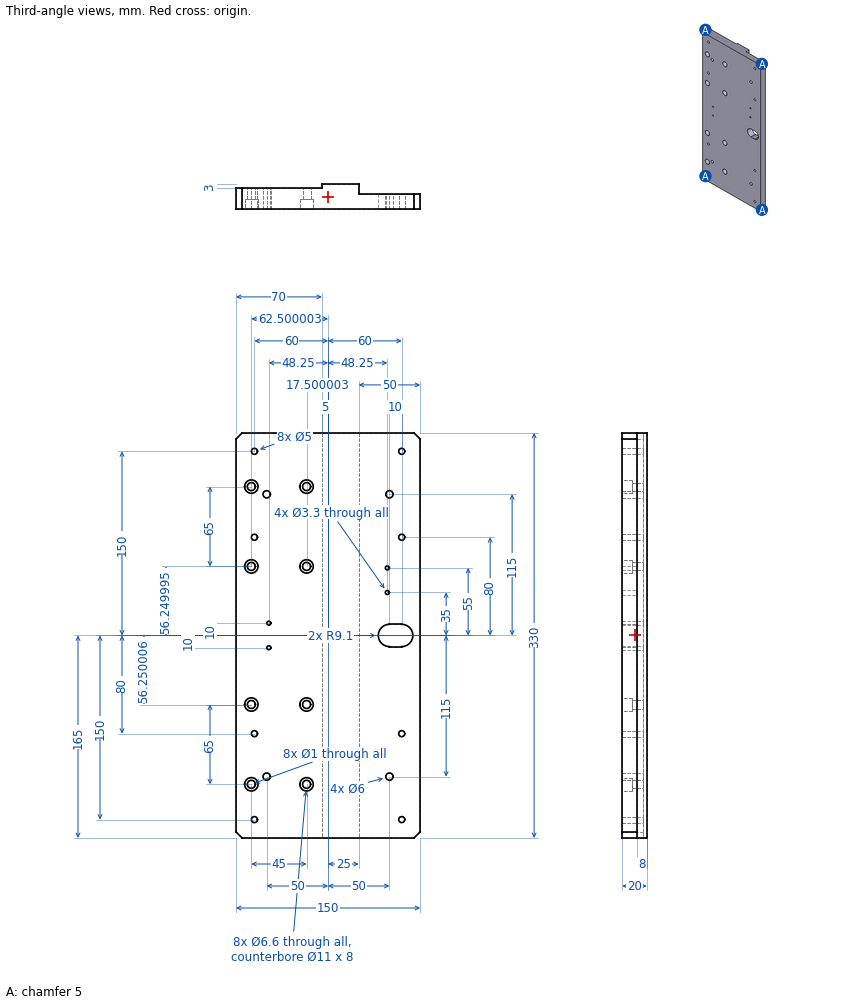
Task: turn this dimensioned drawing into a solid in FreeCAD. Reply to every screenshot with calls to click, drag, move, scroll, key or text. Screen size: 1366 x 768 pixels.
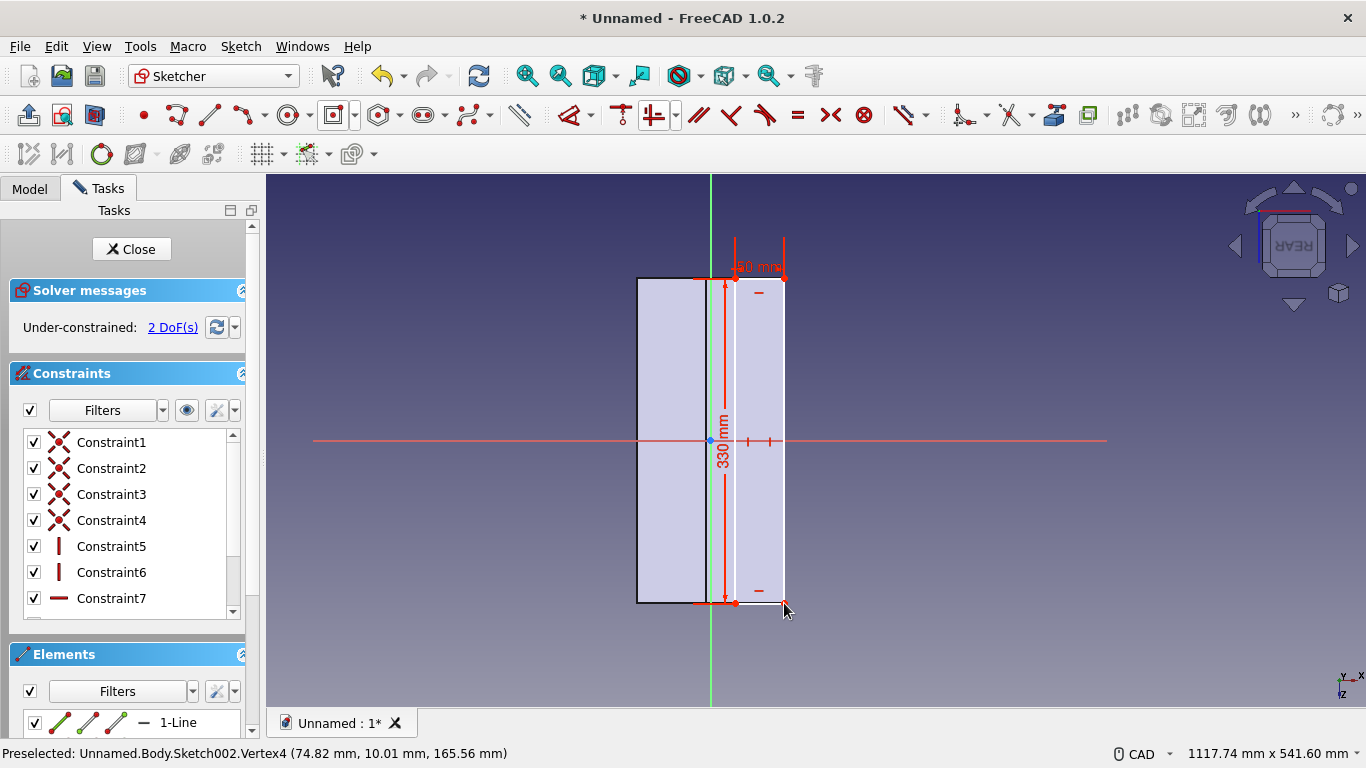
click(568, 116)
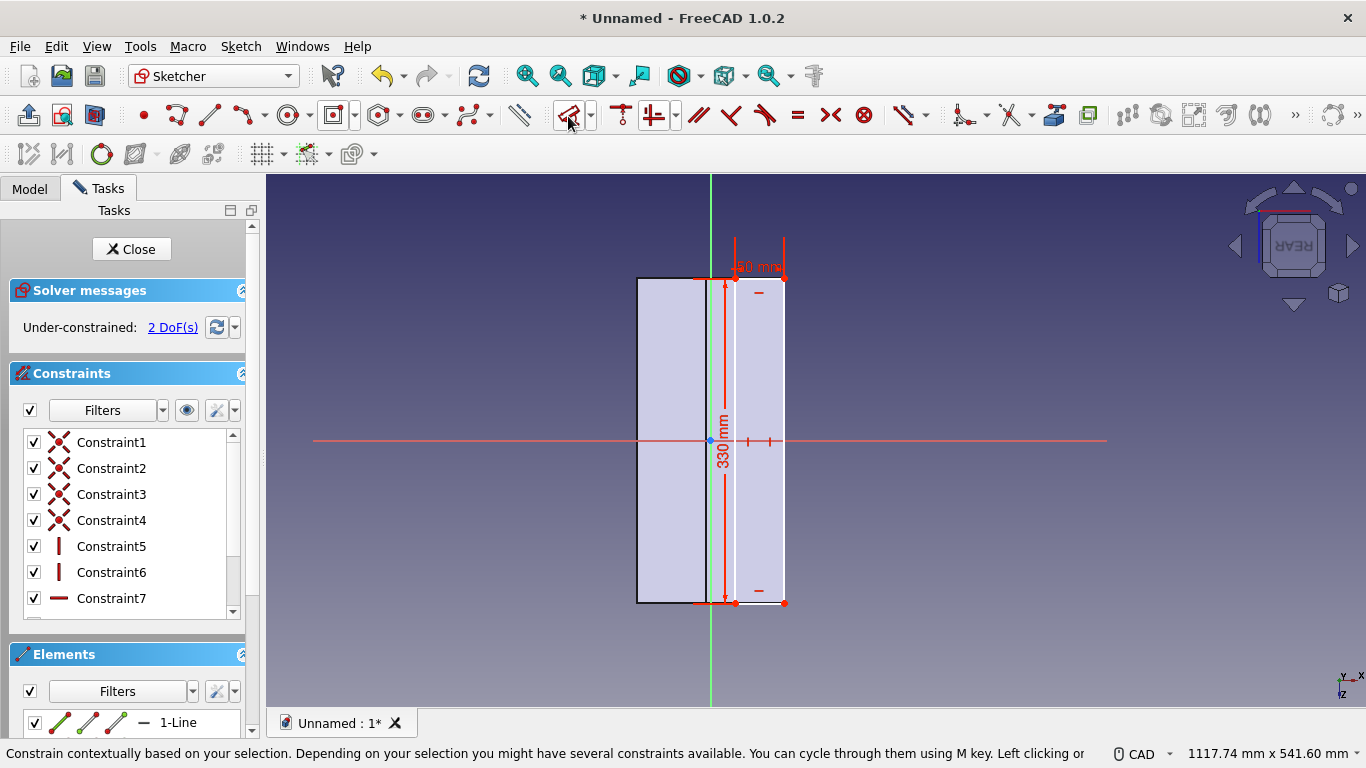
scroll(735, 279, up, 3)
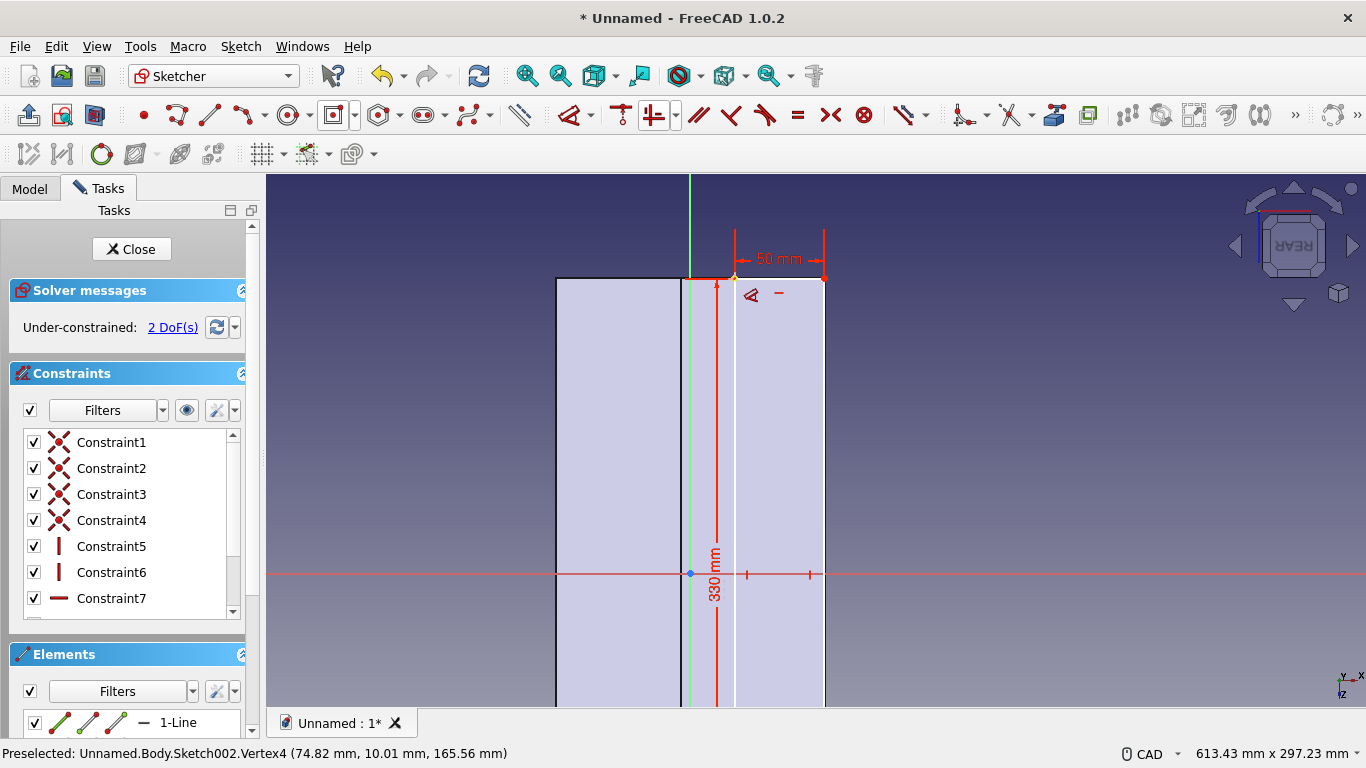
click(735, 279)
click(712, 245)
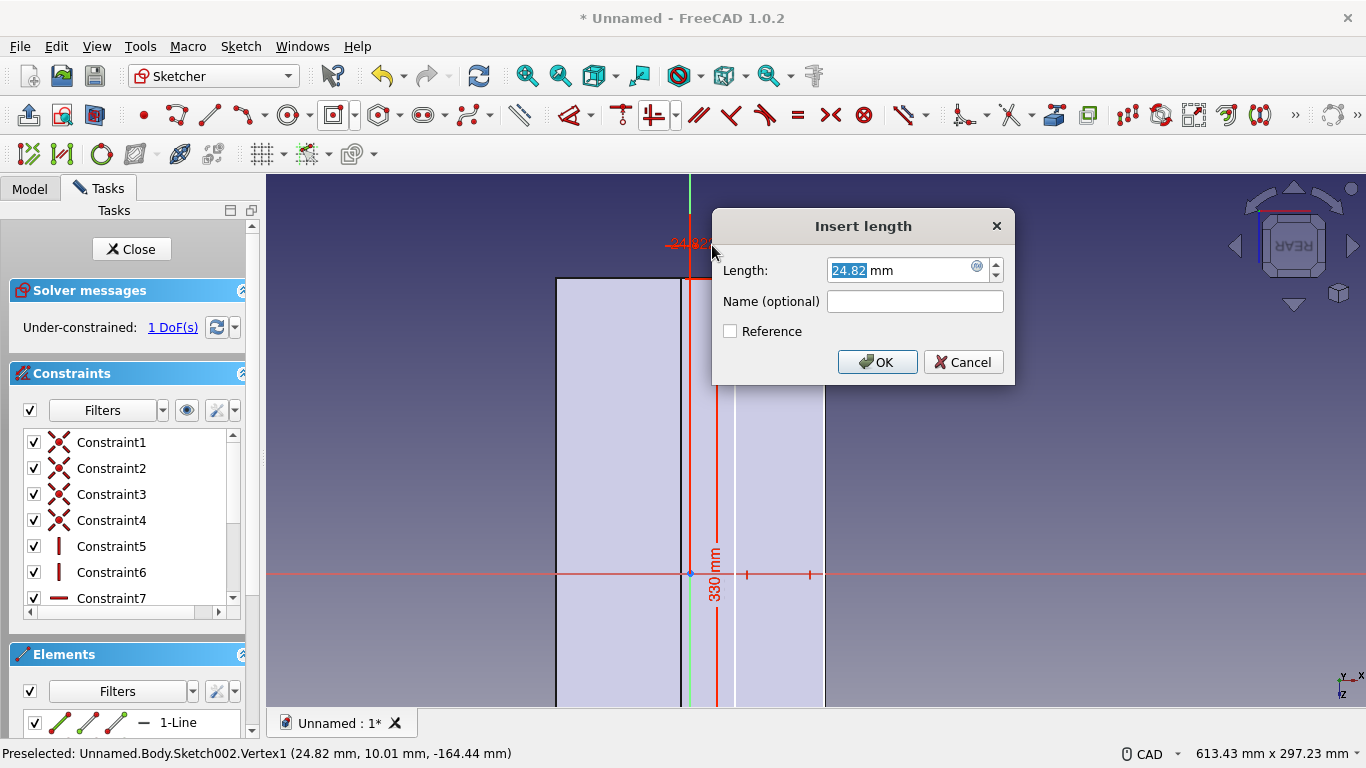
text(25)
key(Return)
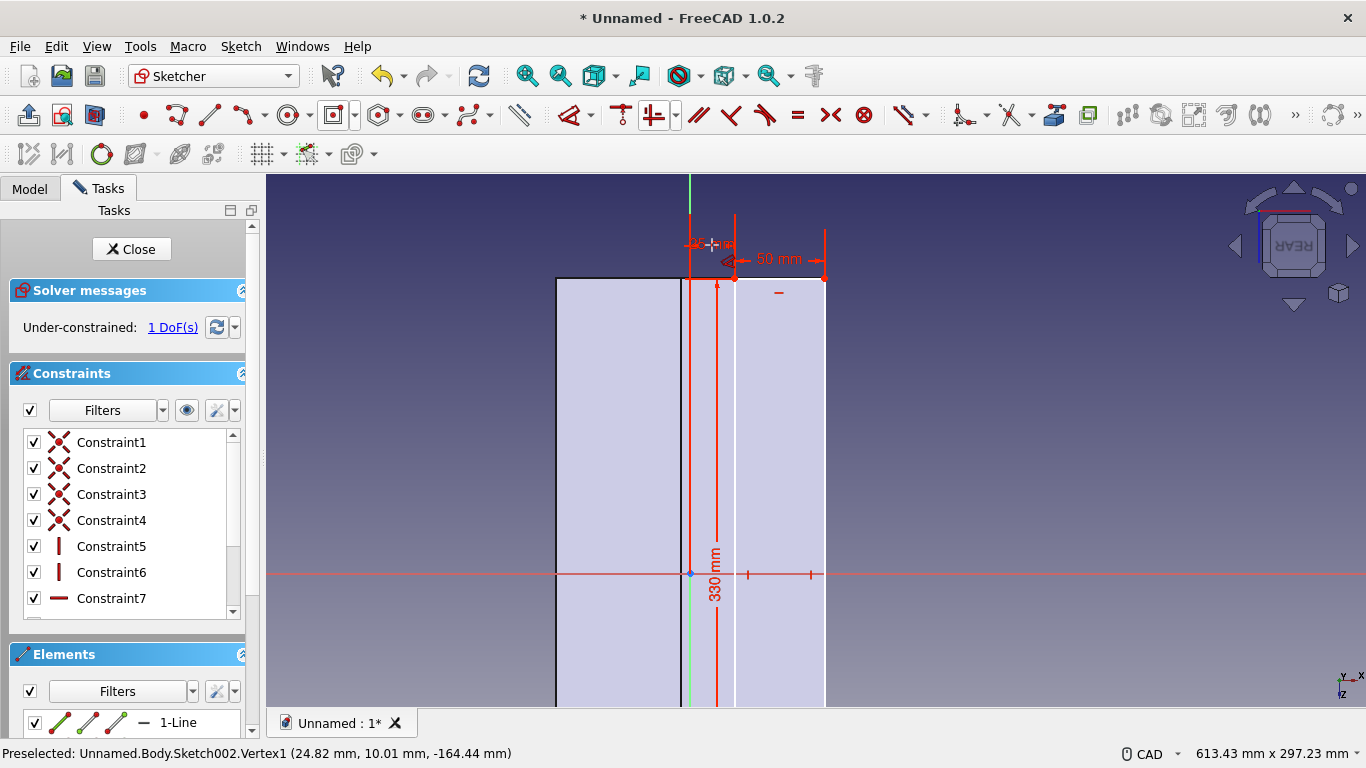
click(735, 279)
click(656, 426)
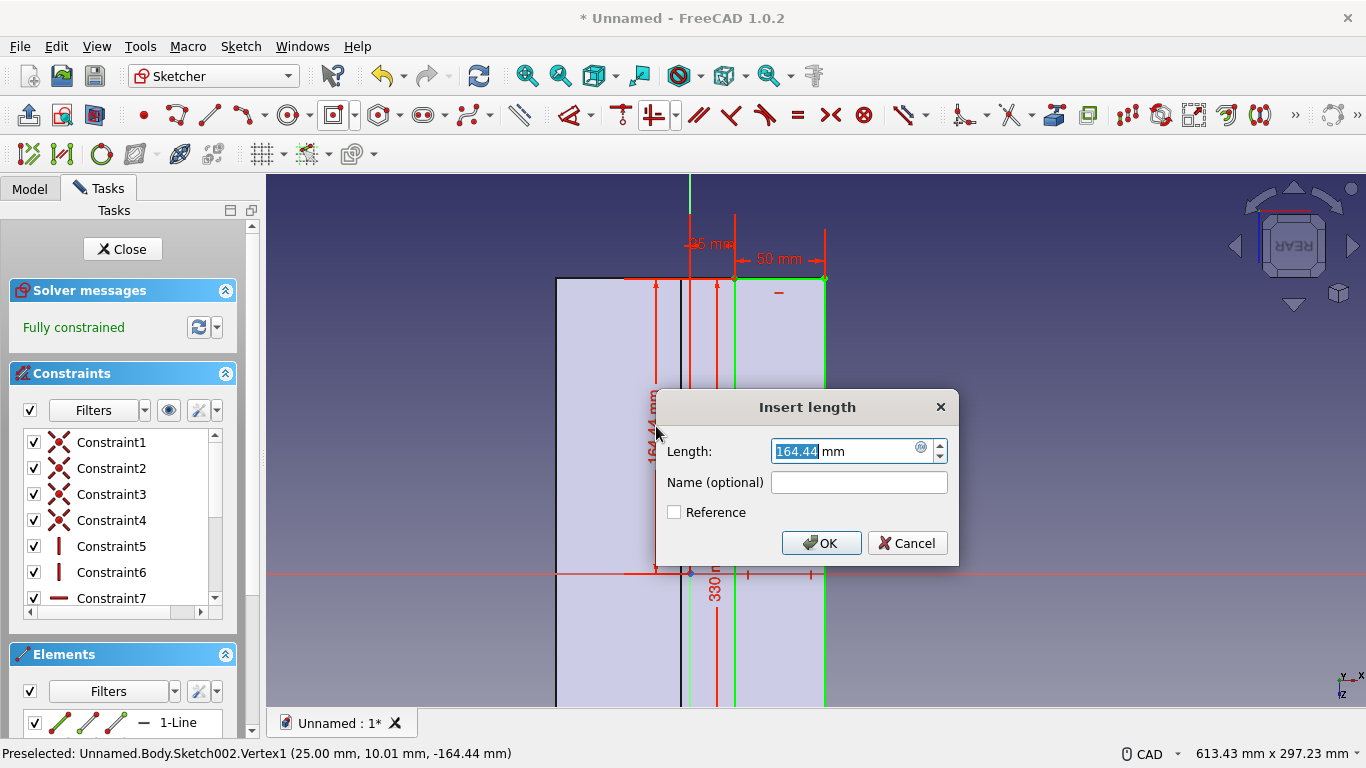
text(165)
key(Return)
key(Escape)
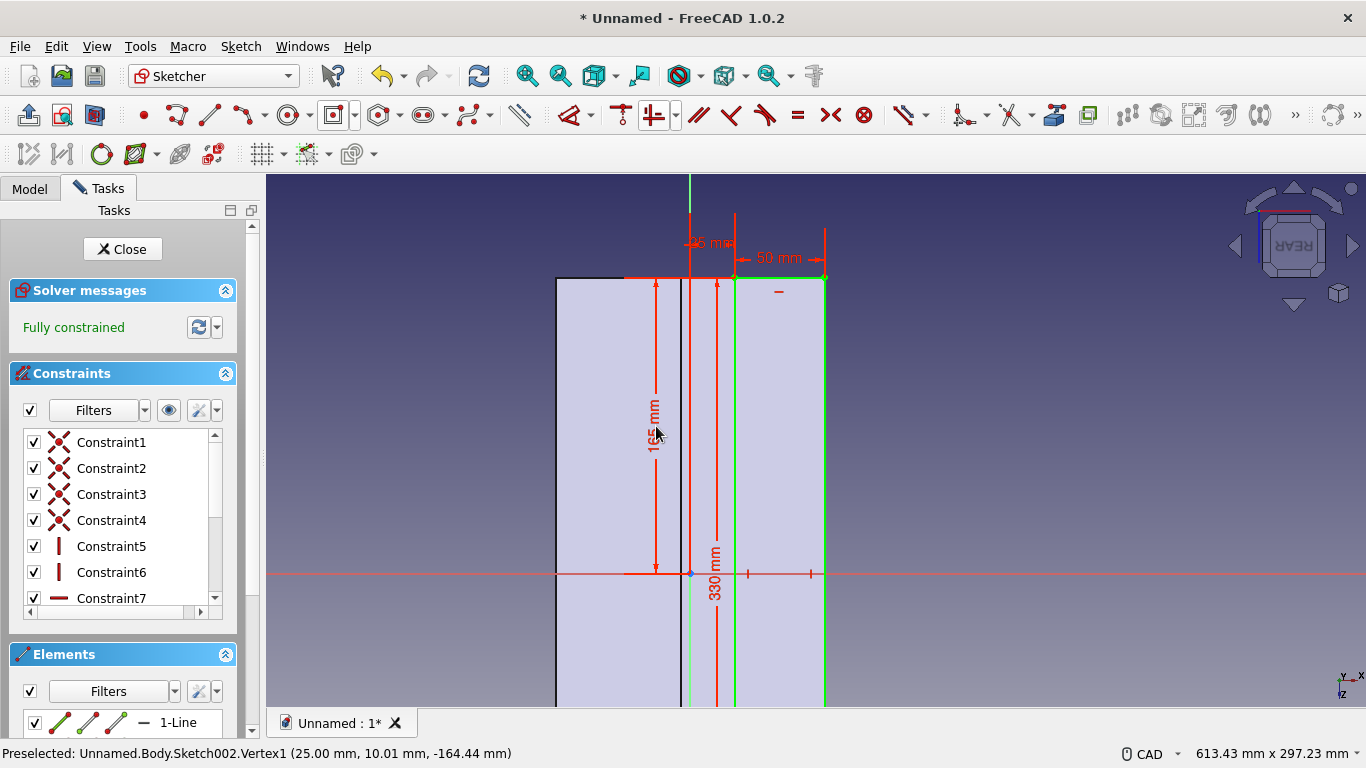
click(123, 249)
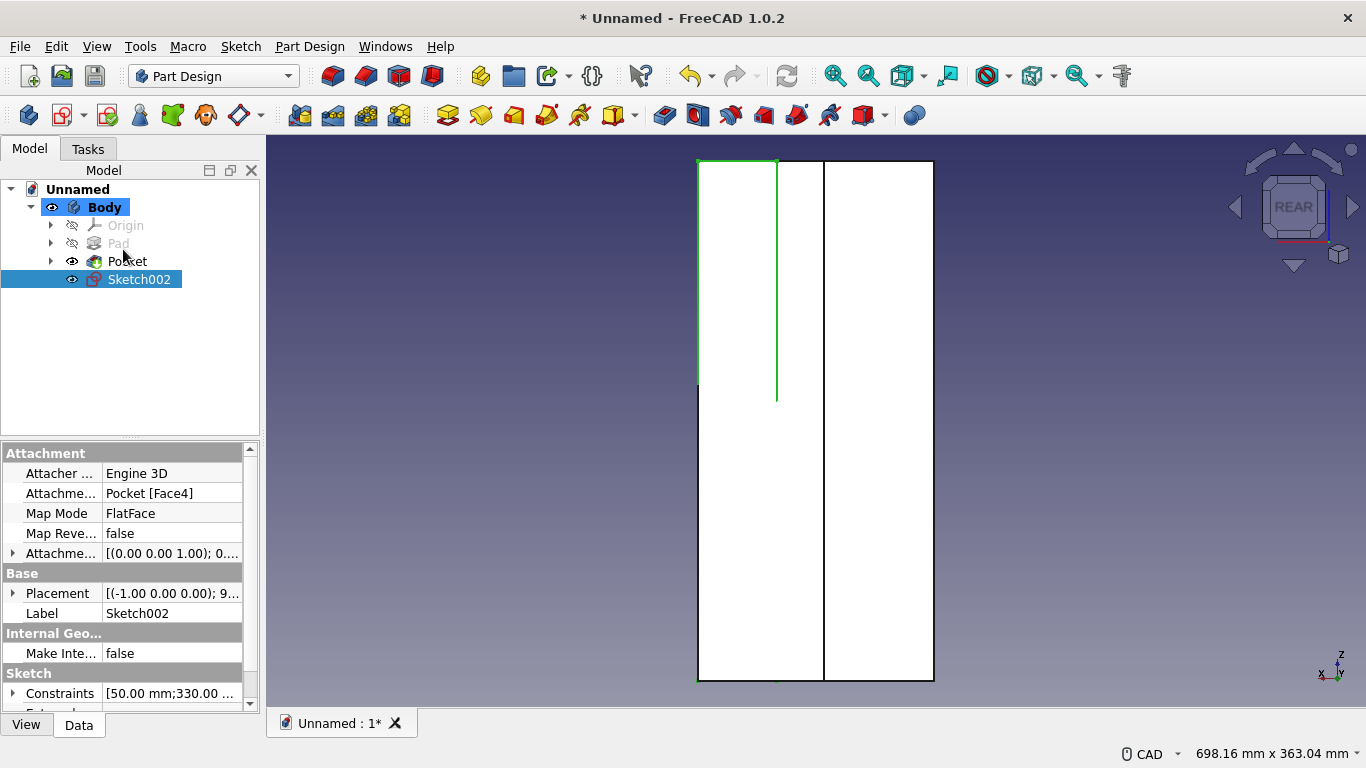
click(665, 116)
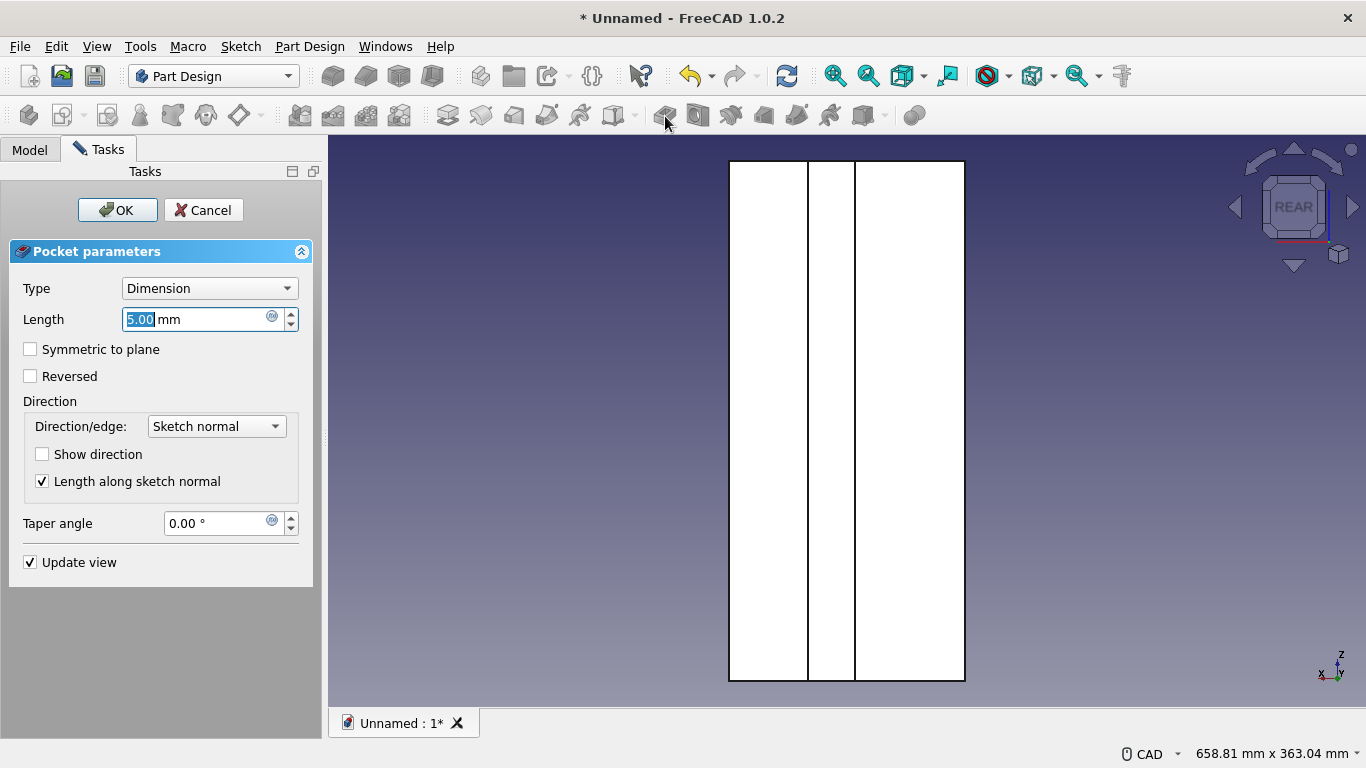
text(8)
key(Tab)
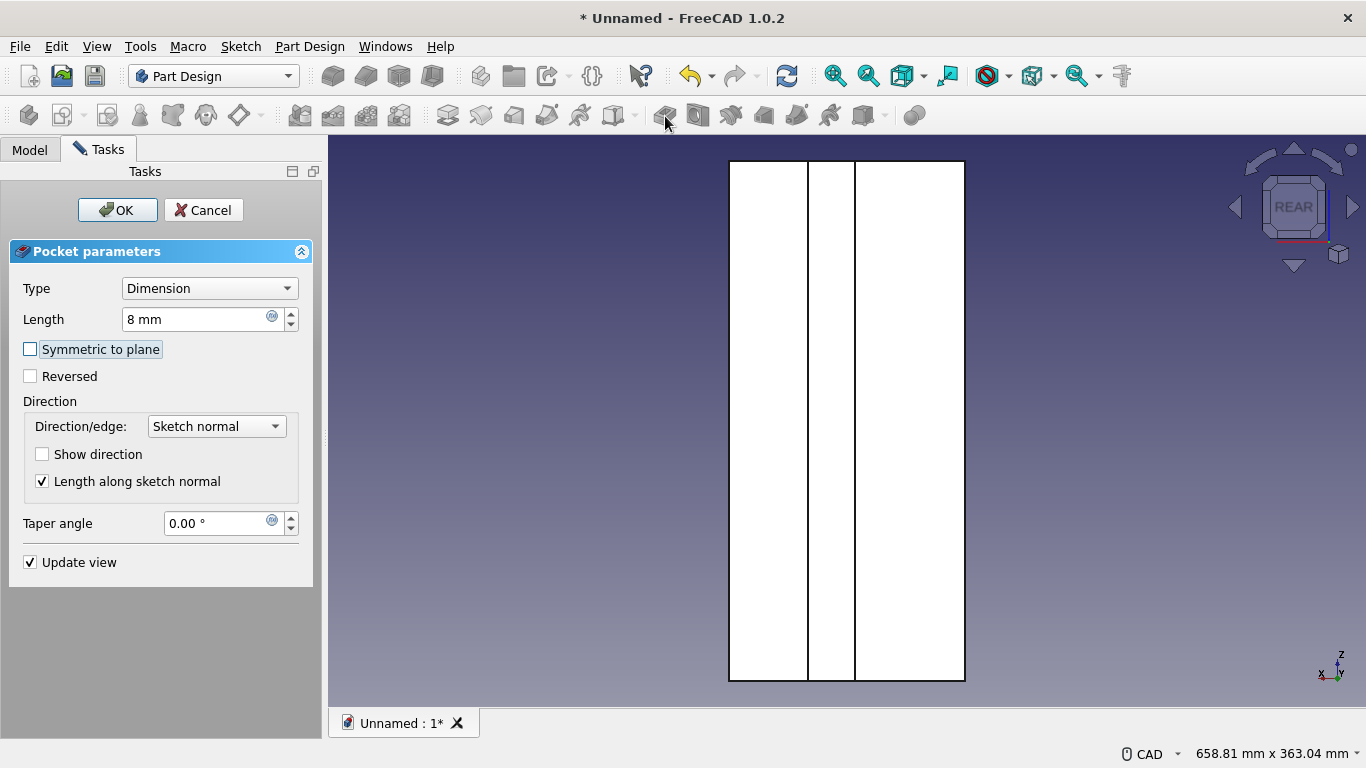
click(118, 210)